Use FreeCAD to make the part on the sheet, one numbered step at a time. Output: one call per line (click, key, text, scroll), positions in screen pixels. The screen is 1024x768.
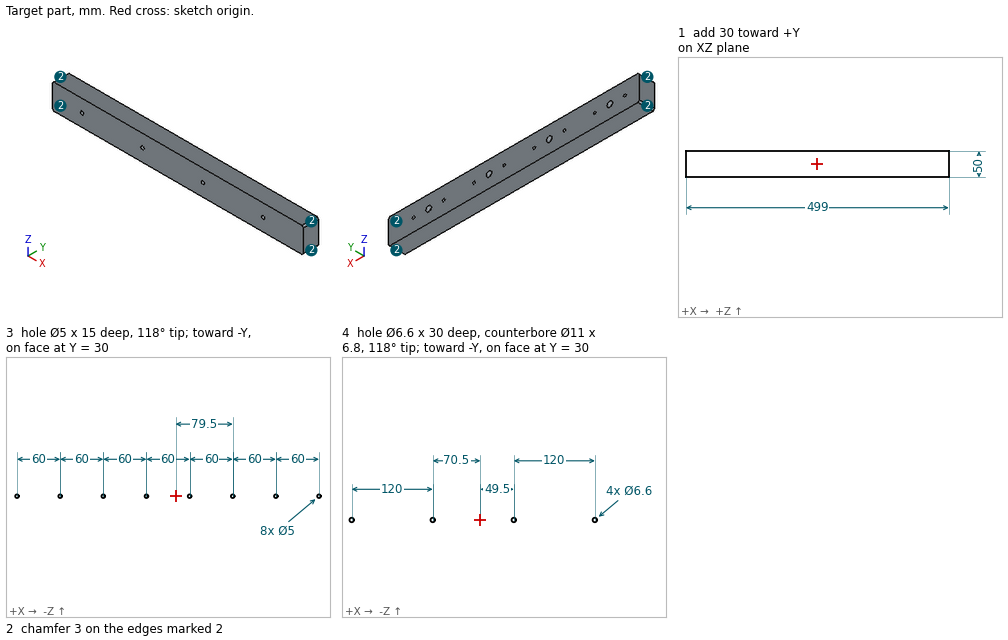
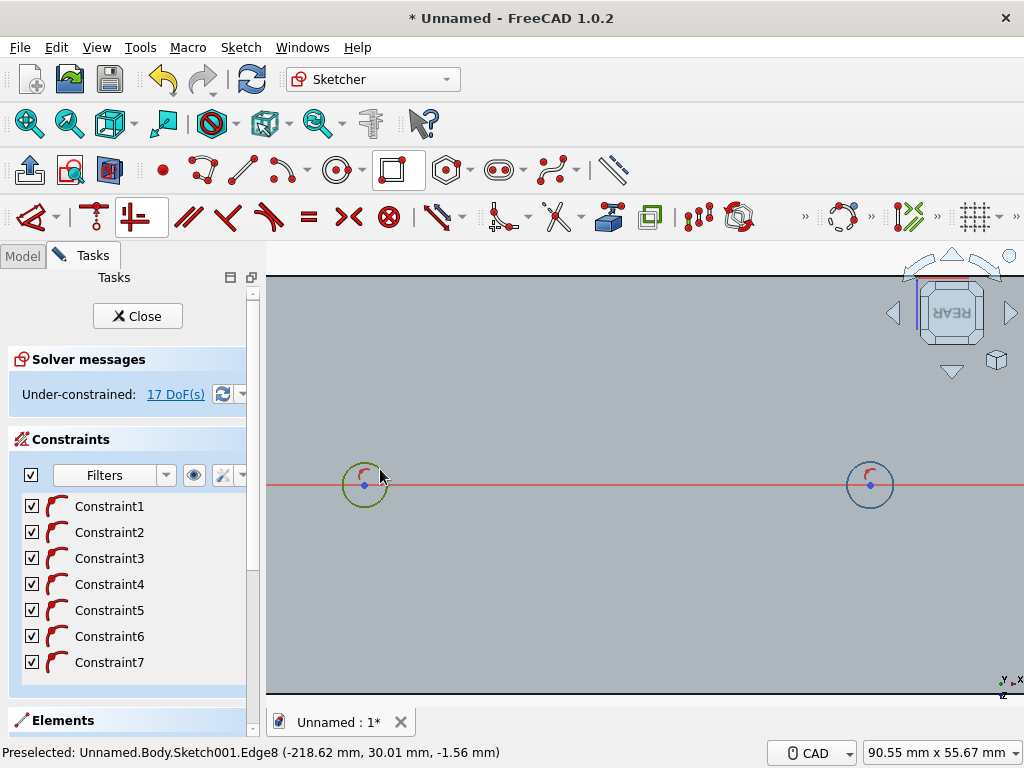
click(310, 218)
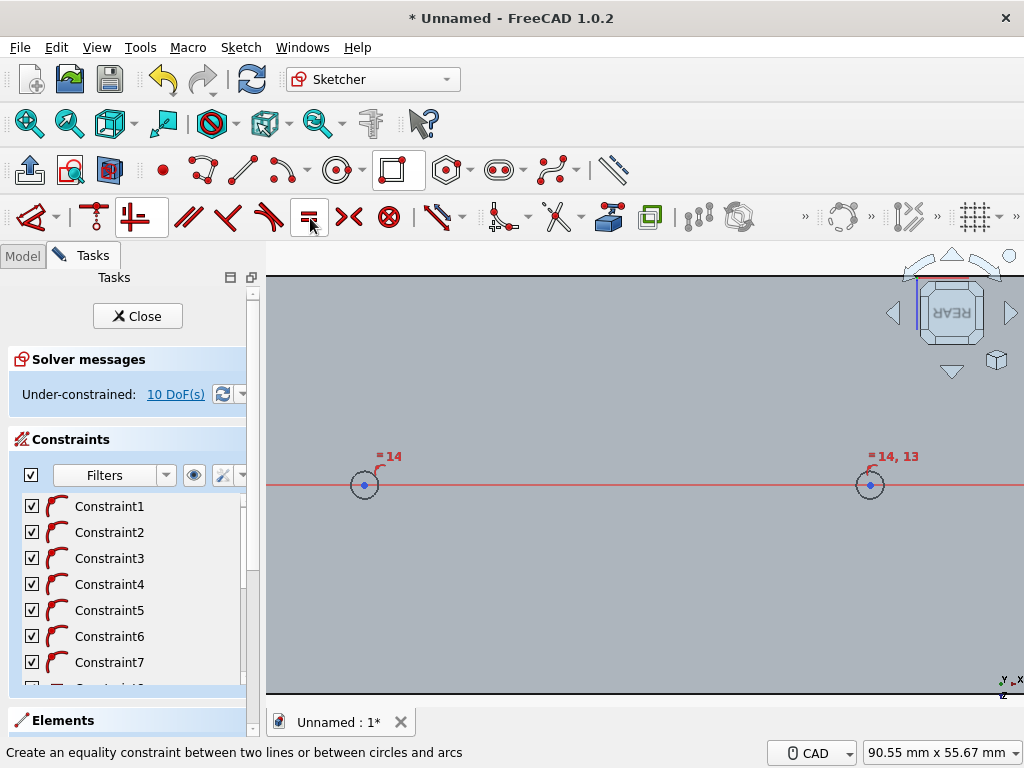
scroll(384, 473, down, 11)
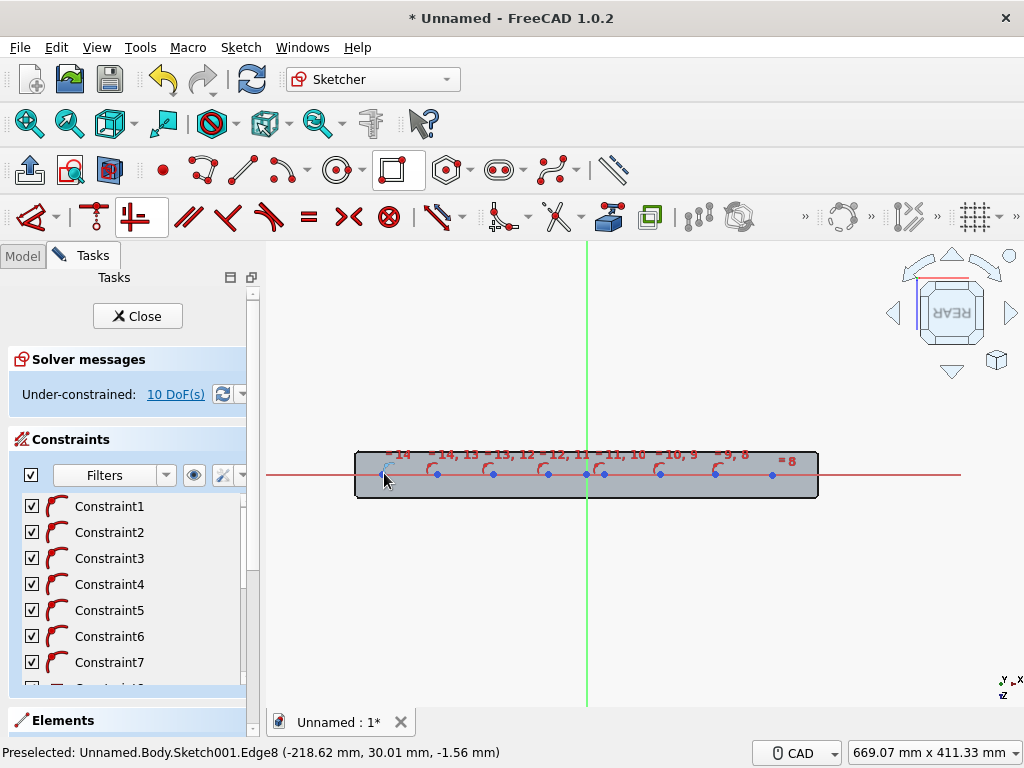
click(772, 476)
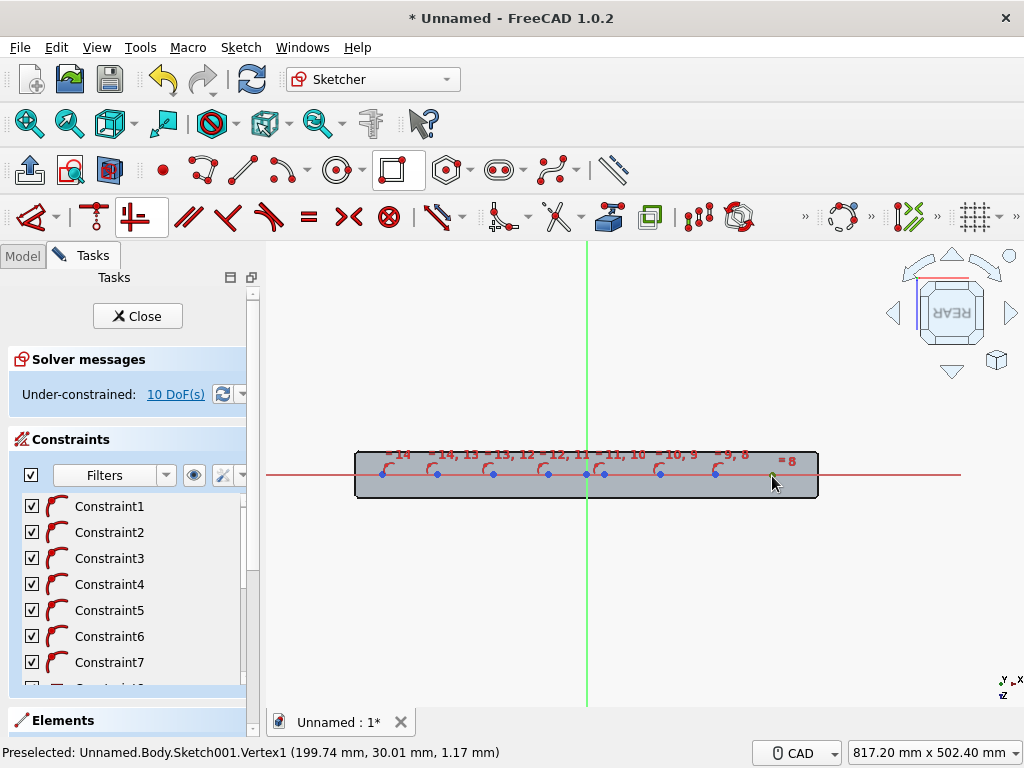
click(334, 475)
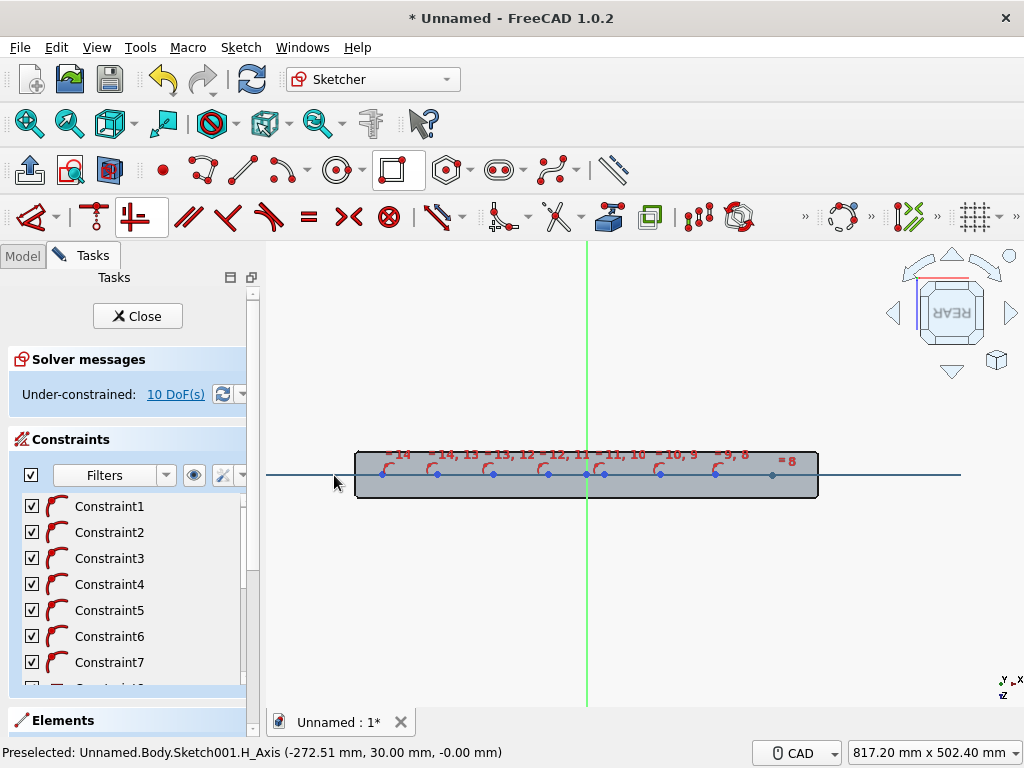
click(94, 218)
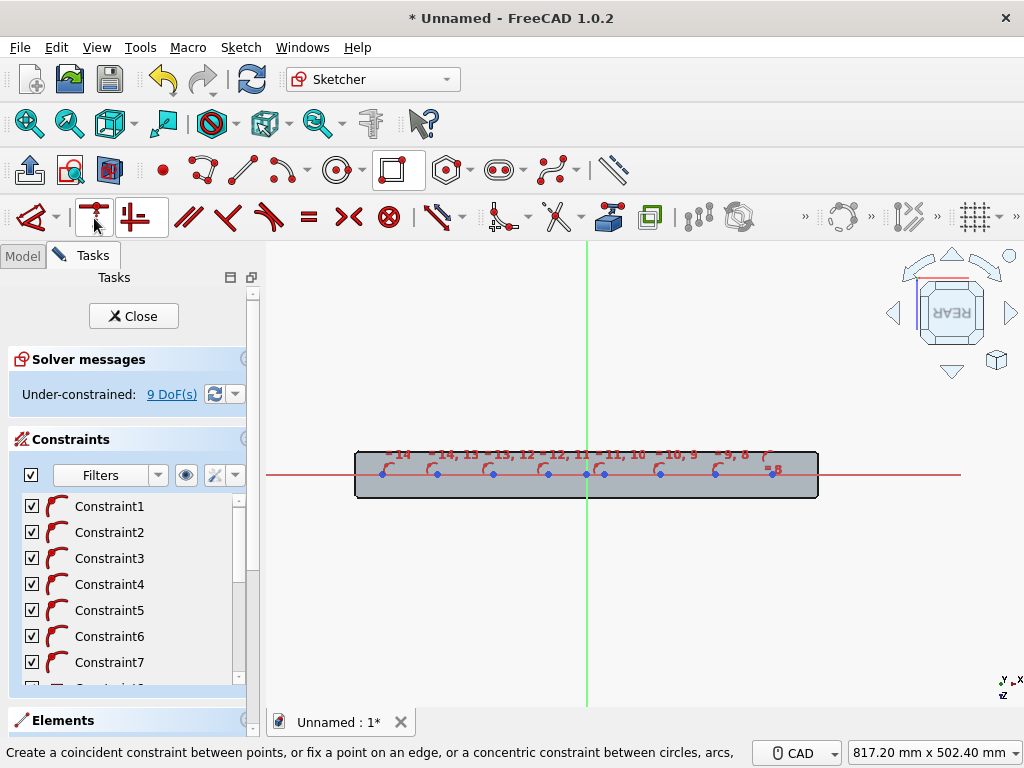
click(32, 218)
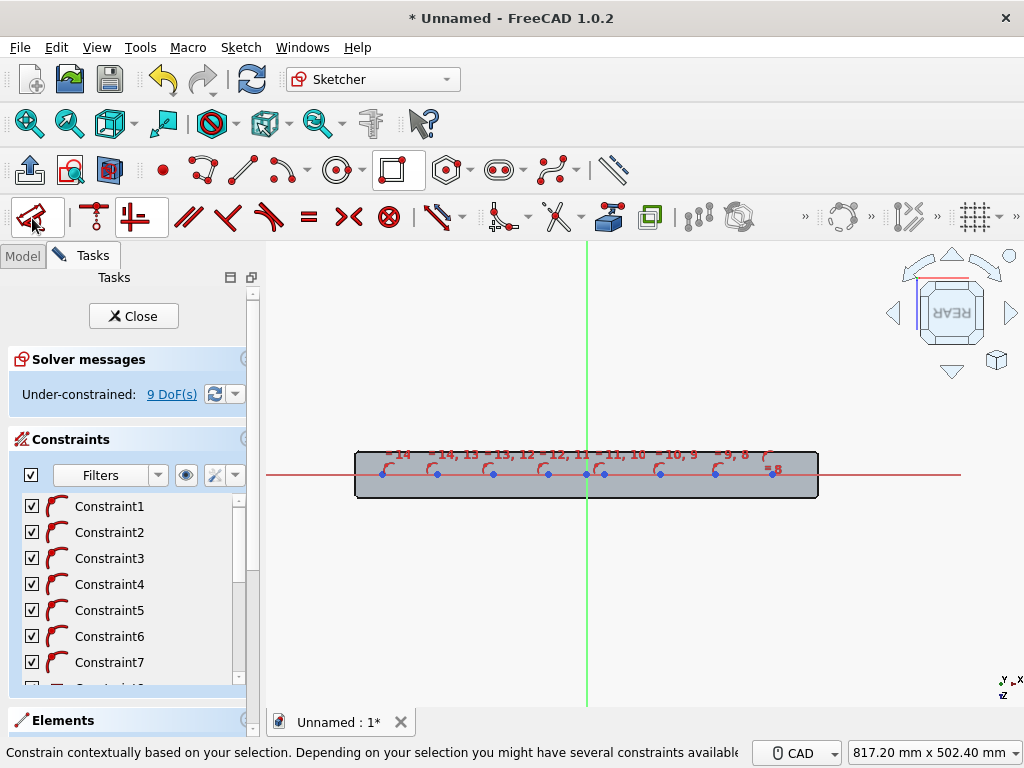
scroll(771, 474, up, 12)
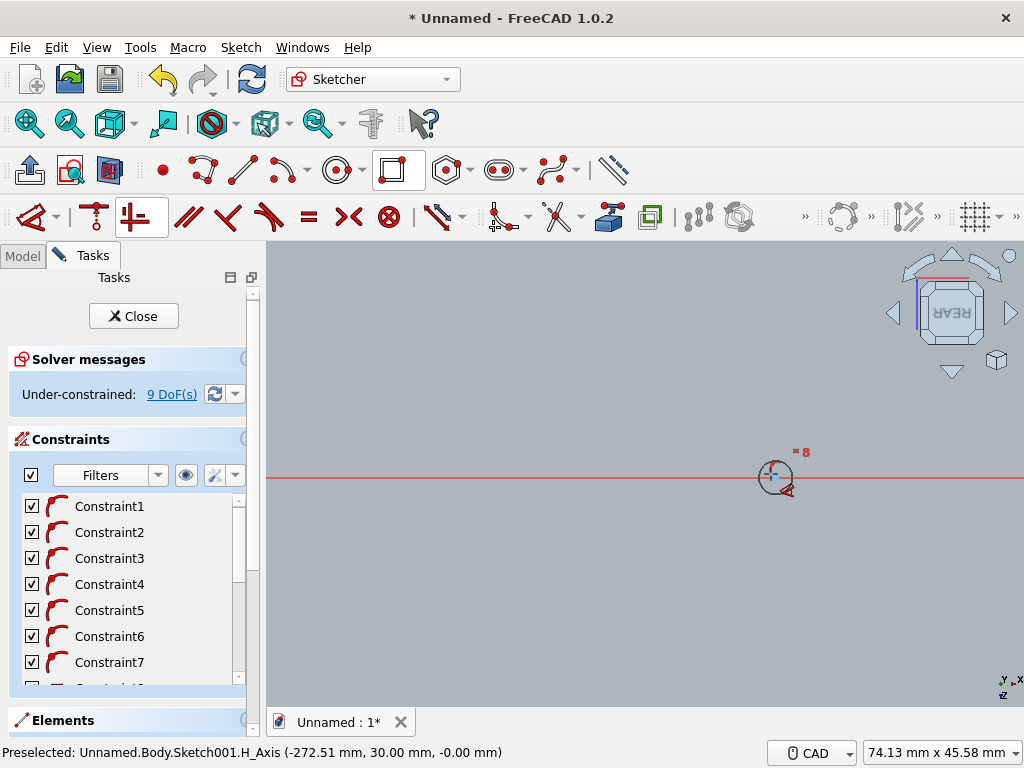
click(764, 466)
click(741, 443)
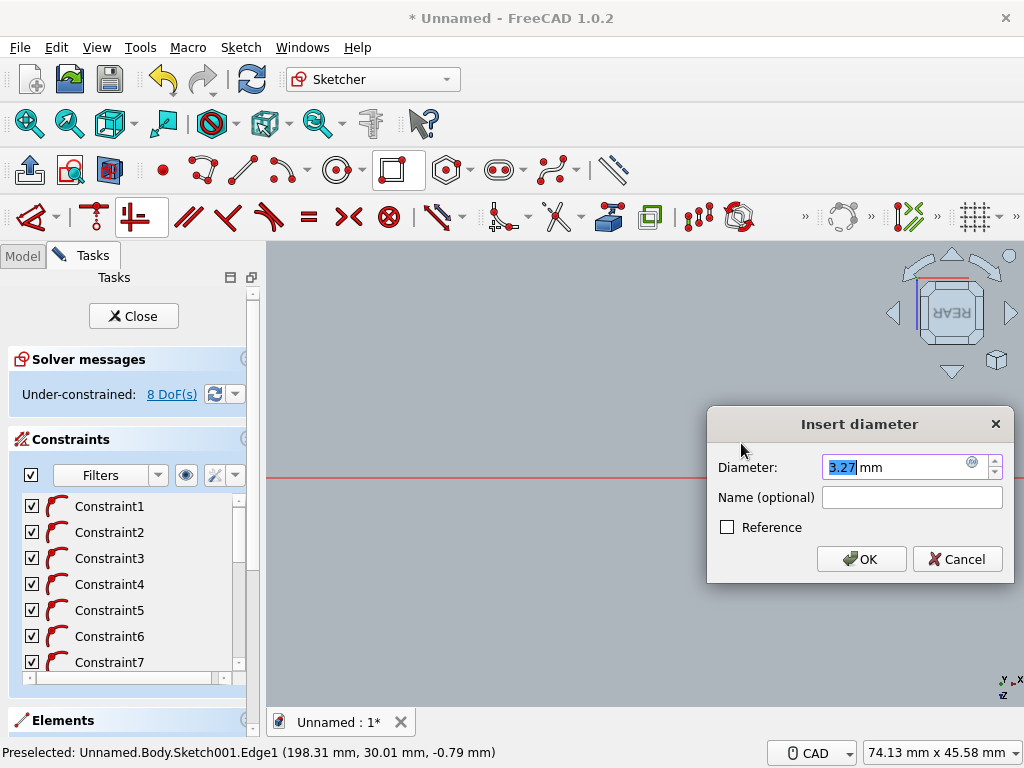
text(5)
key(Return)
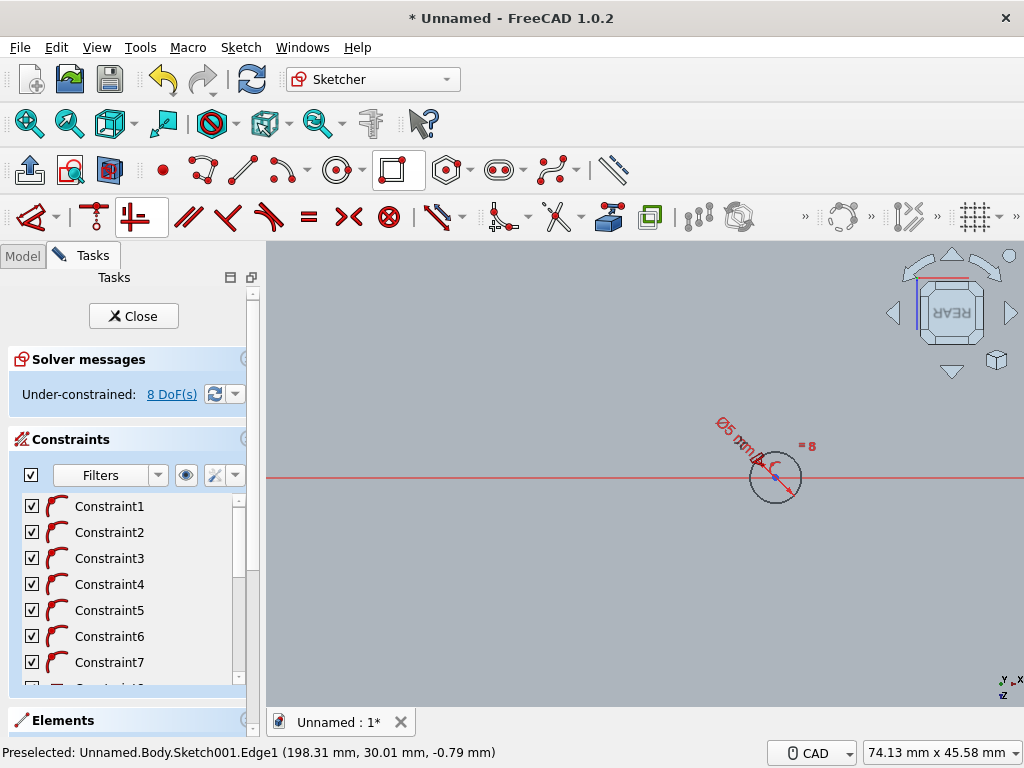
scroll(771, 474, down, 12)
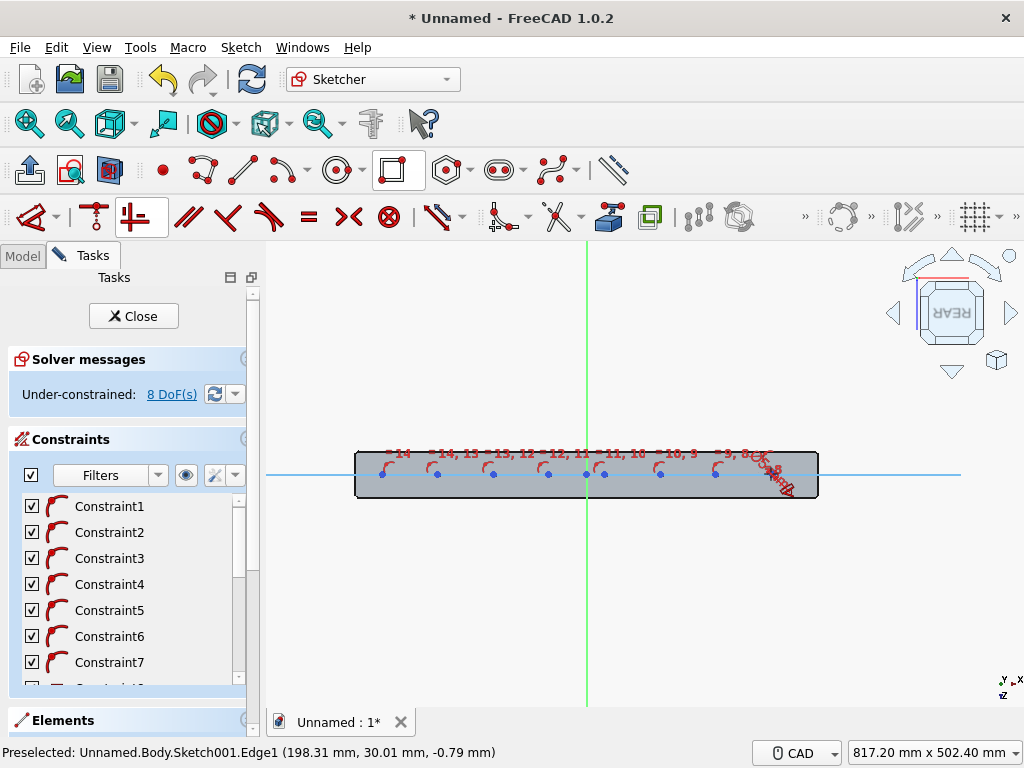
click(772, 475)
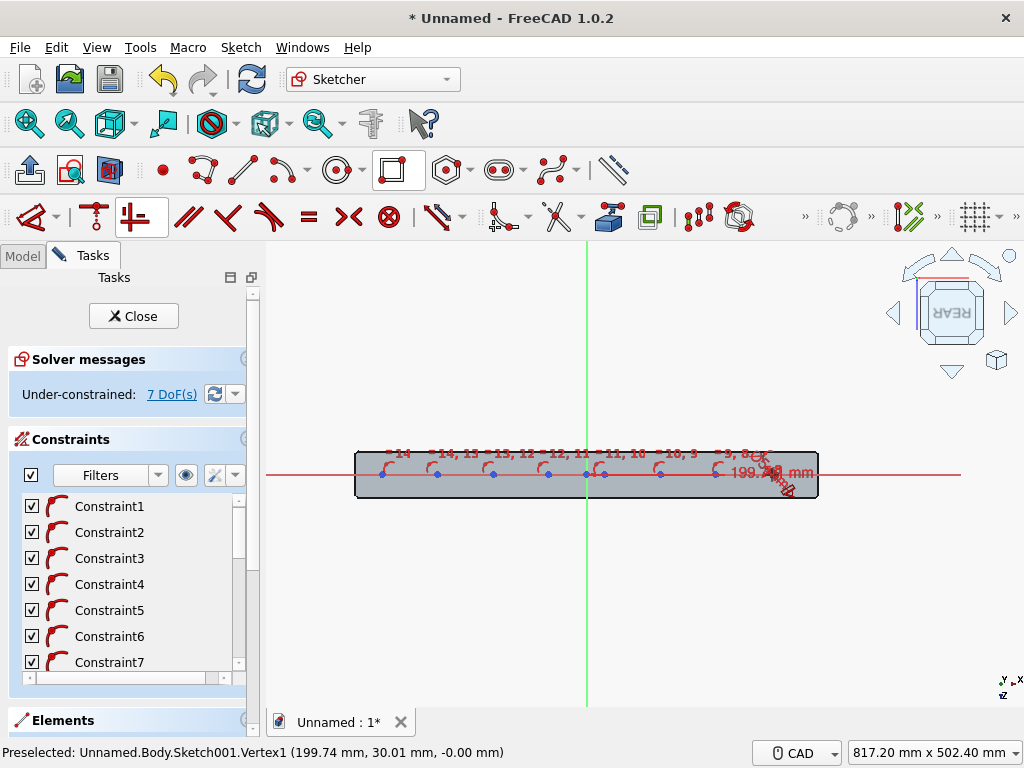
click(716, 475)
click(744, 509)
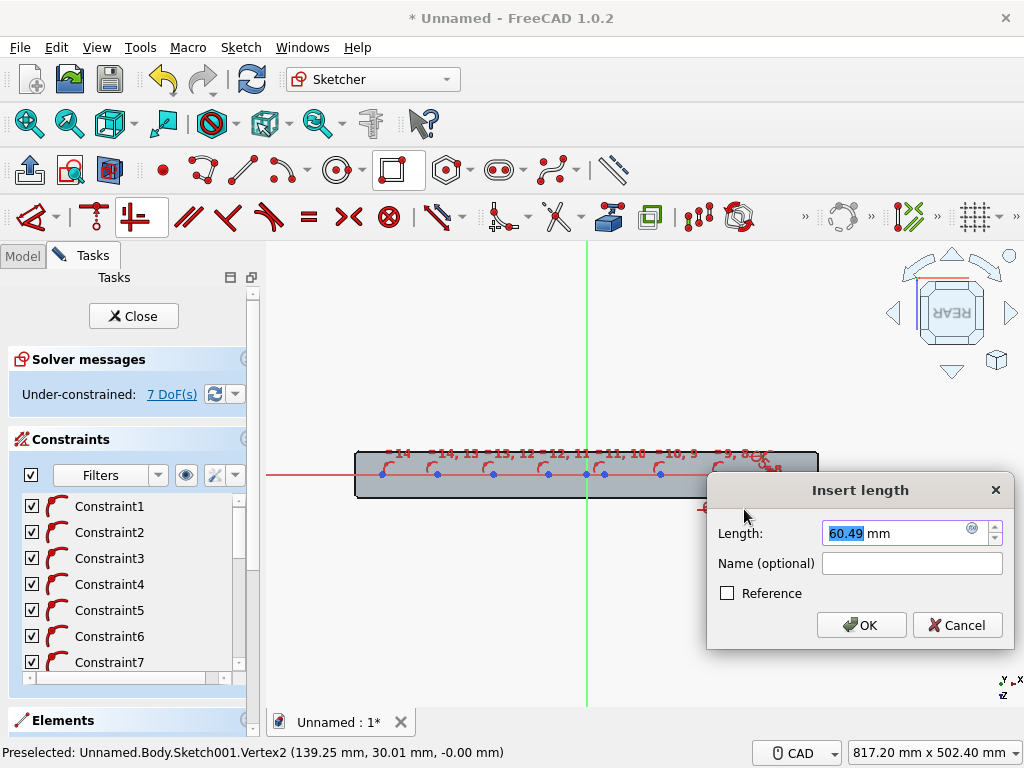
text(60)
key(Return)